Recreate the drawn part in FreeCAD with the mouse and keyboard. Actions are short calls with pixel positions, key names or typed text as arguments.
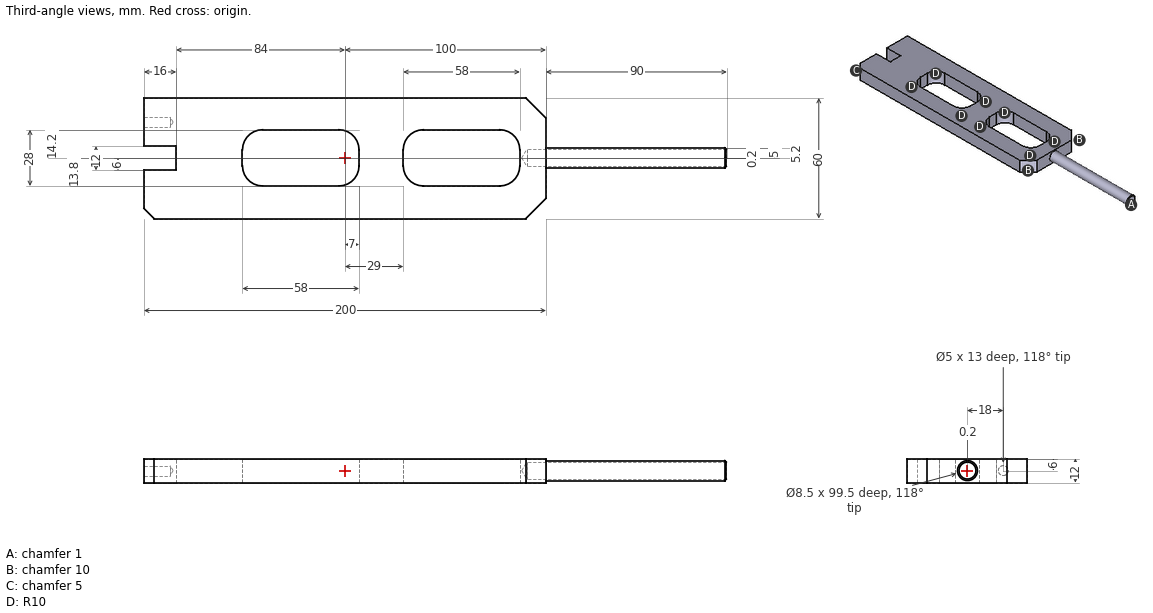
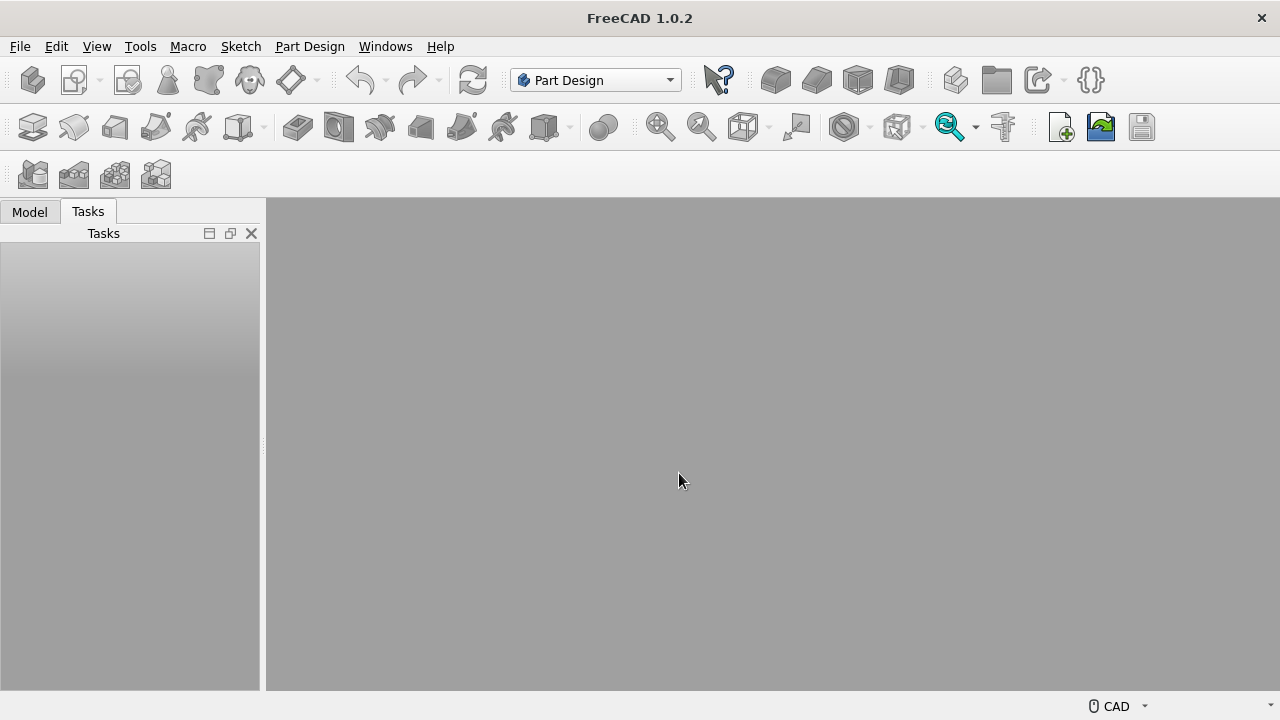
key(ctrl+n)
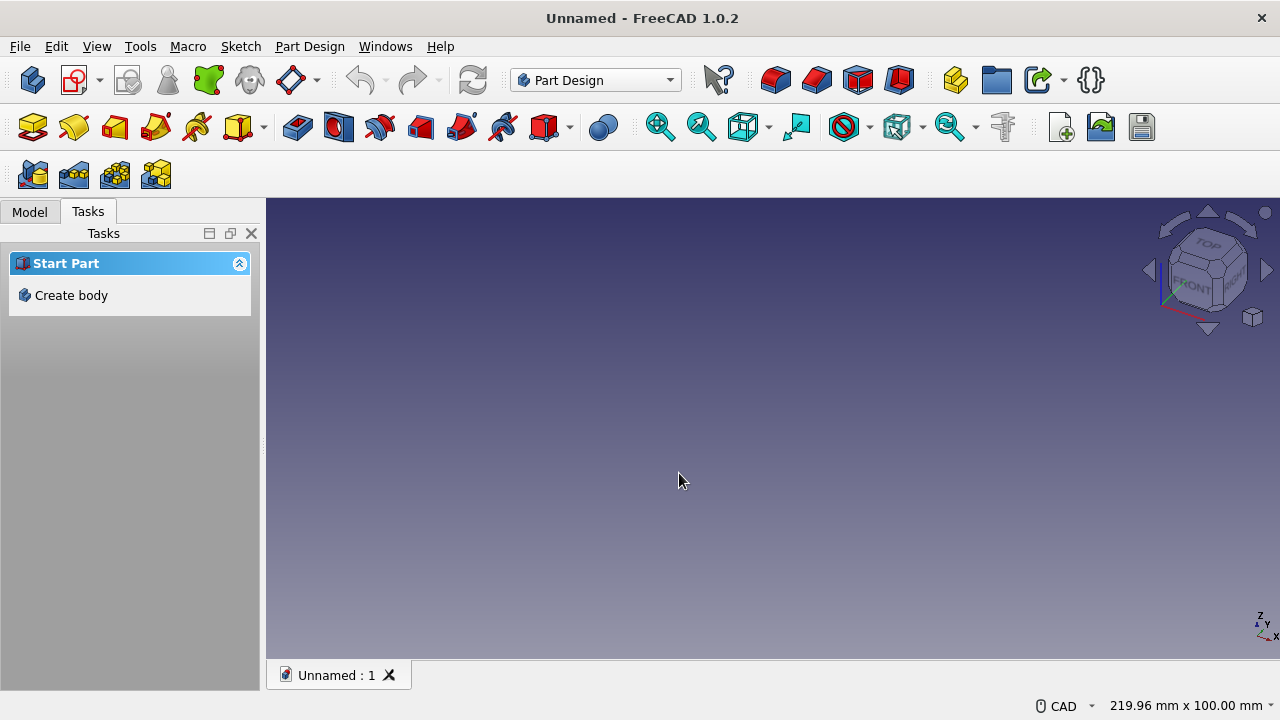
click(33, 80)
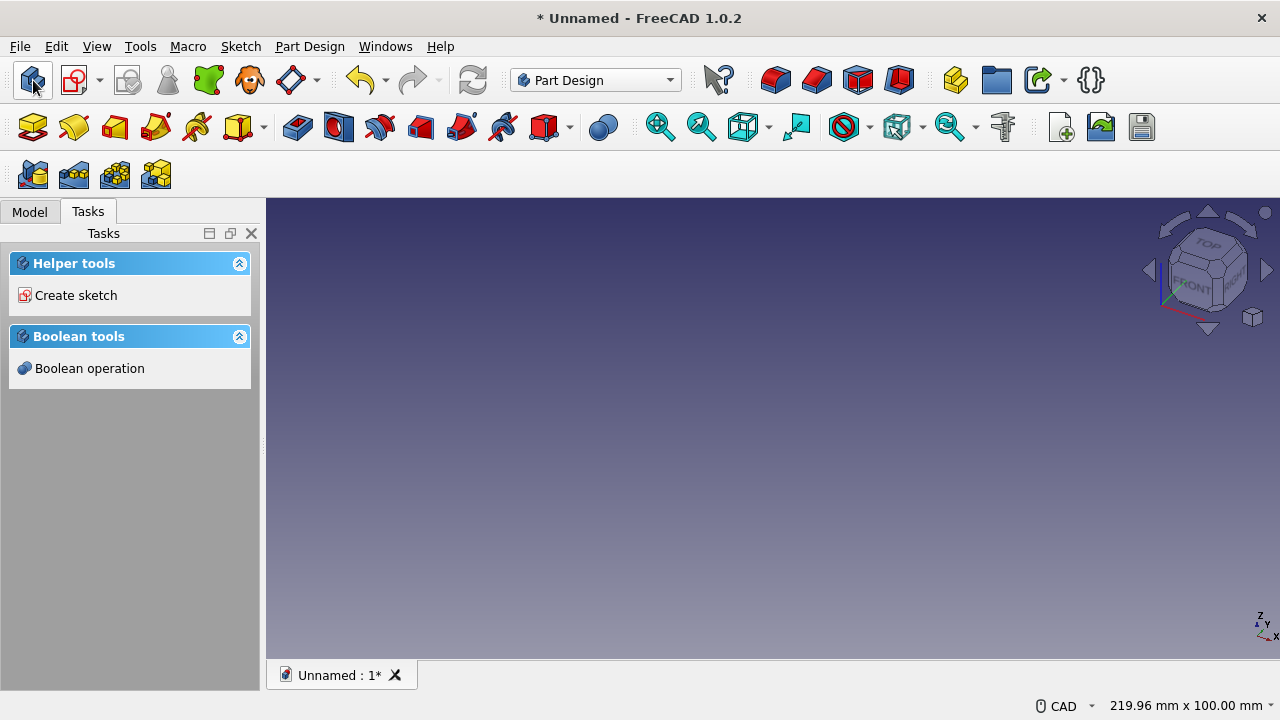
click(30, 212)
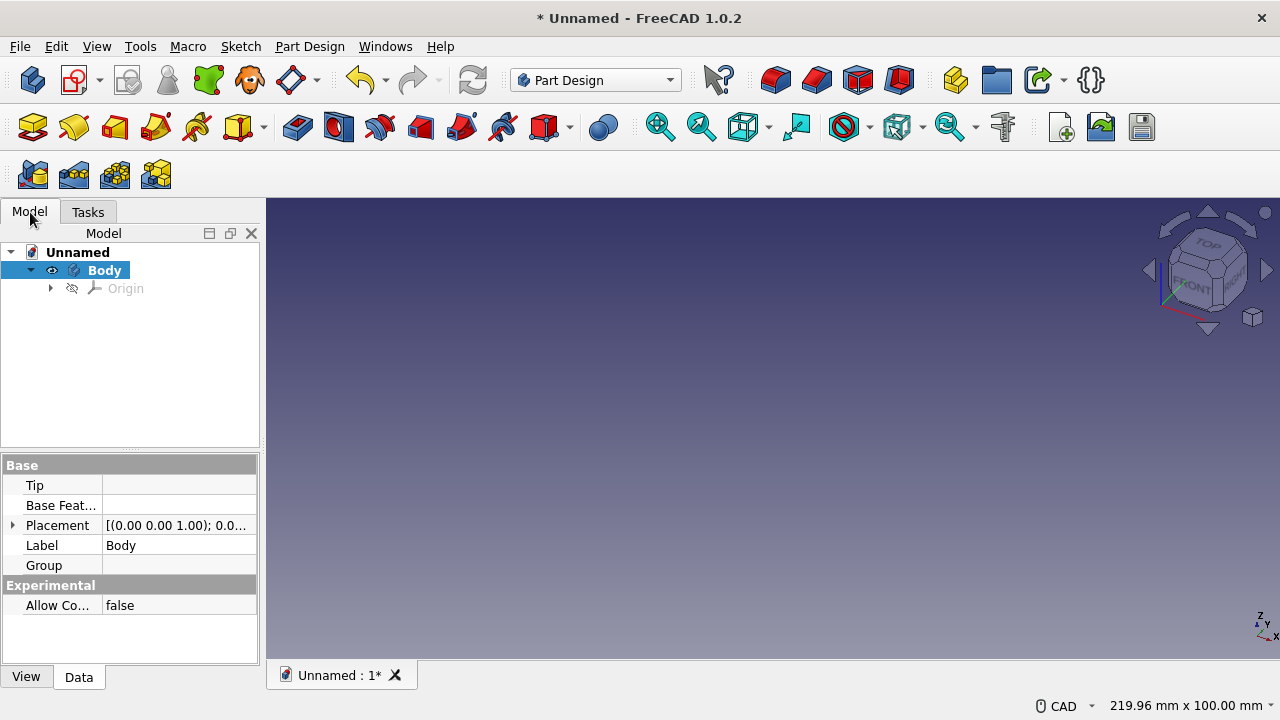
click(51, 288)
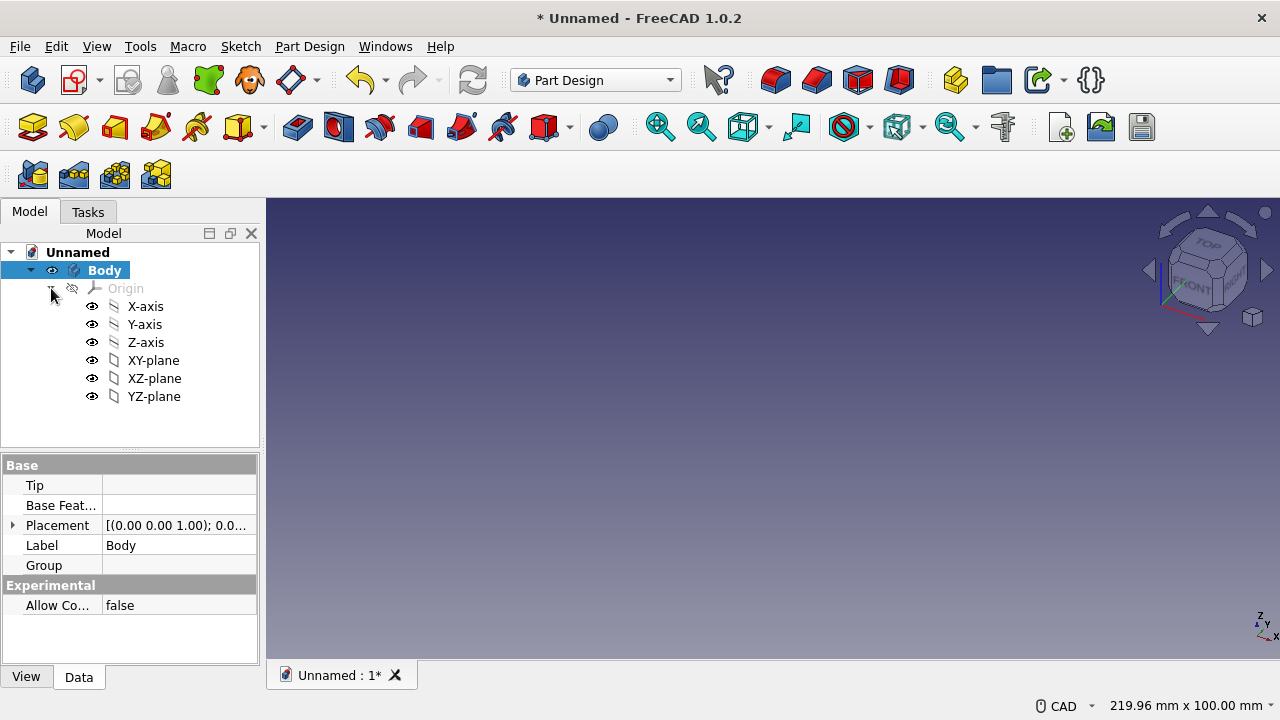
click(137, 360)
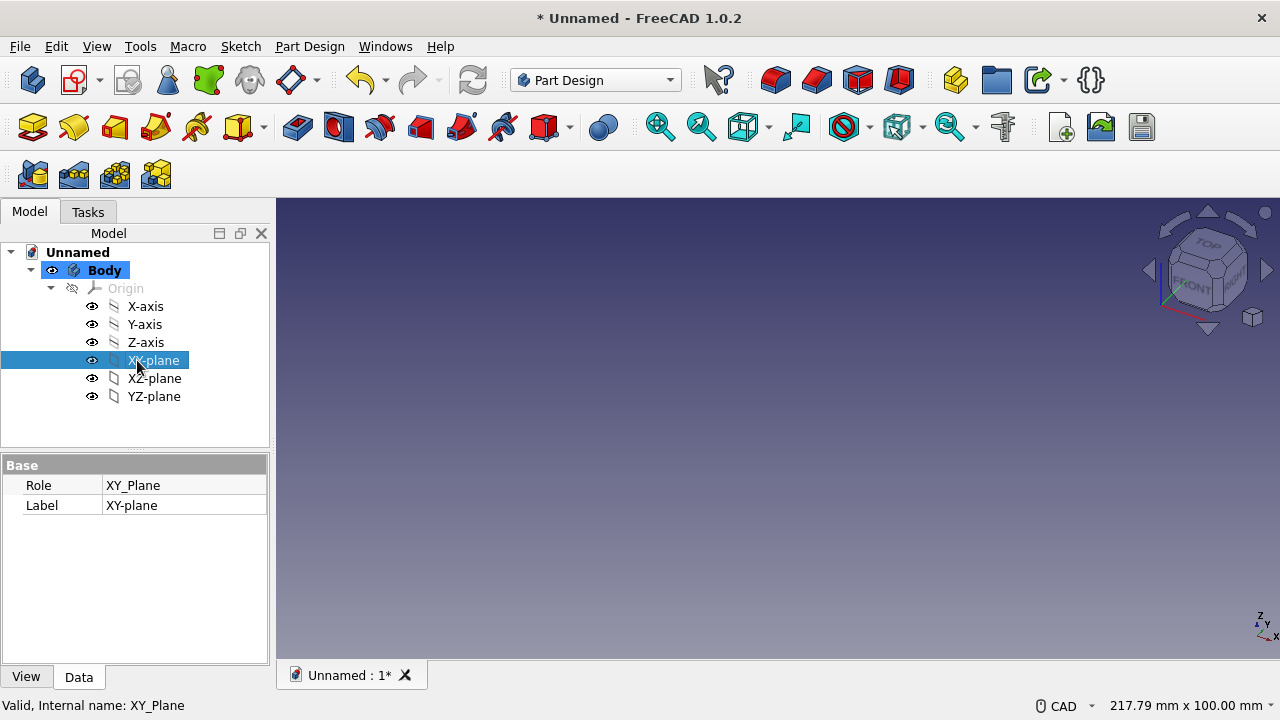
click(290, 80)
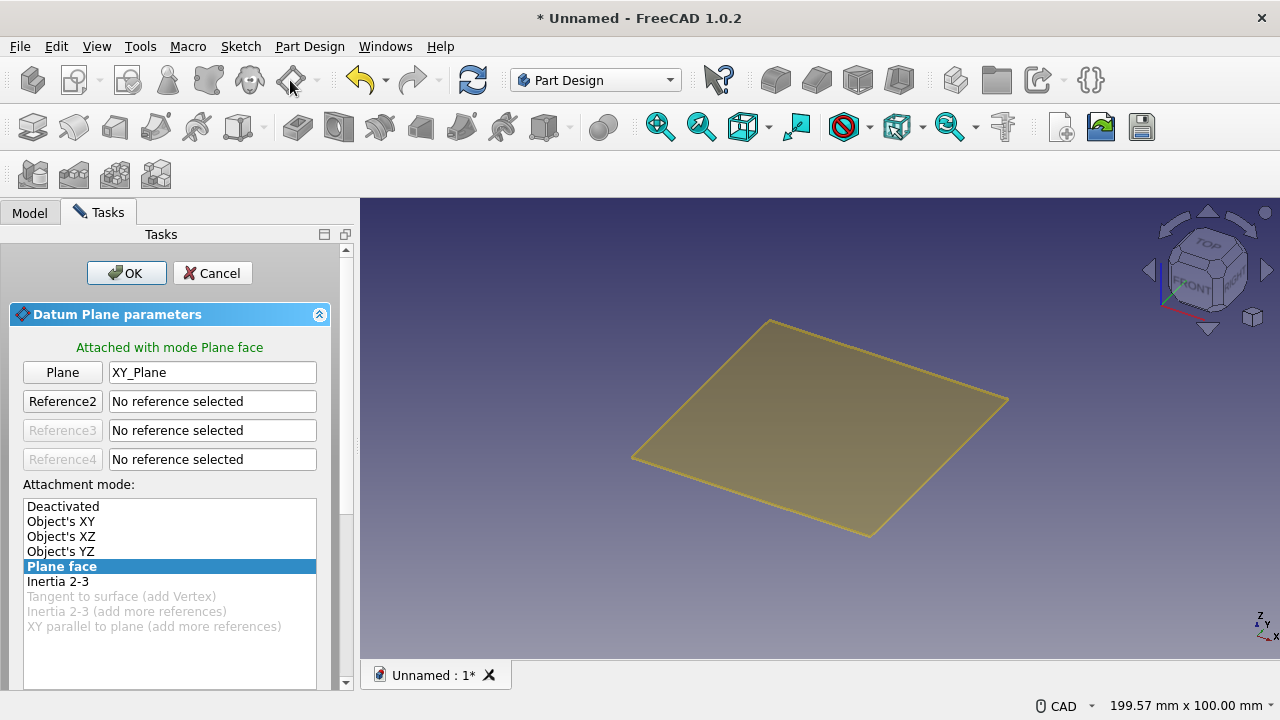
scroll(346, 467, down, 4)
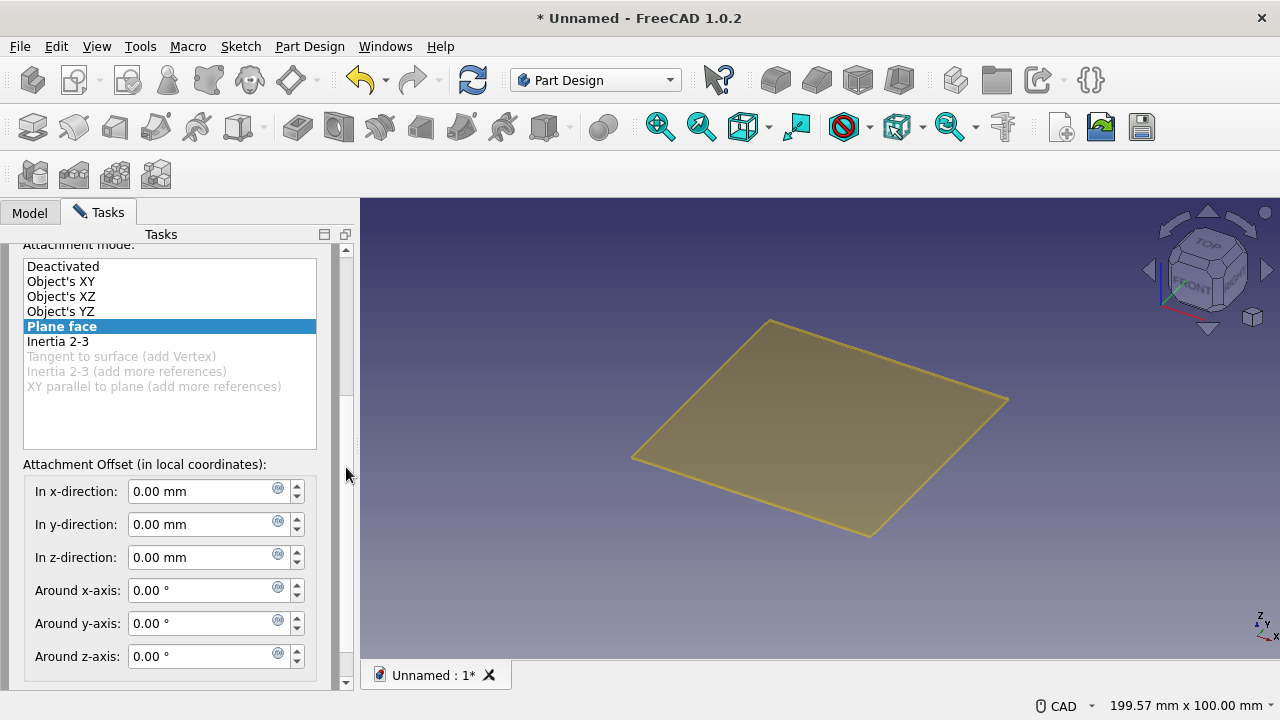
triple_click(210, 558)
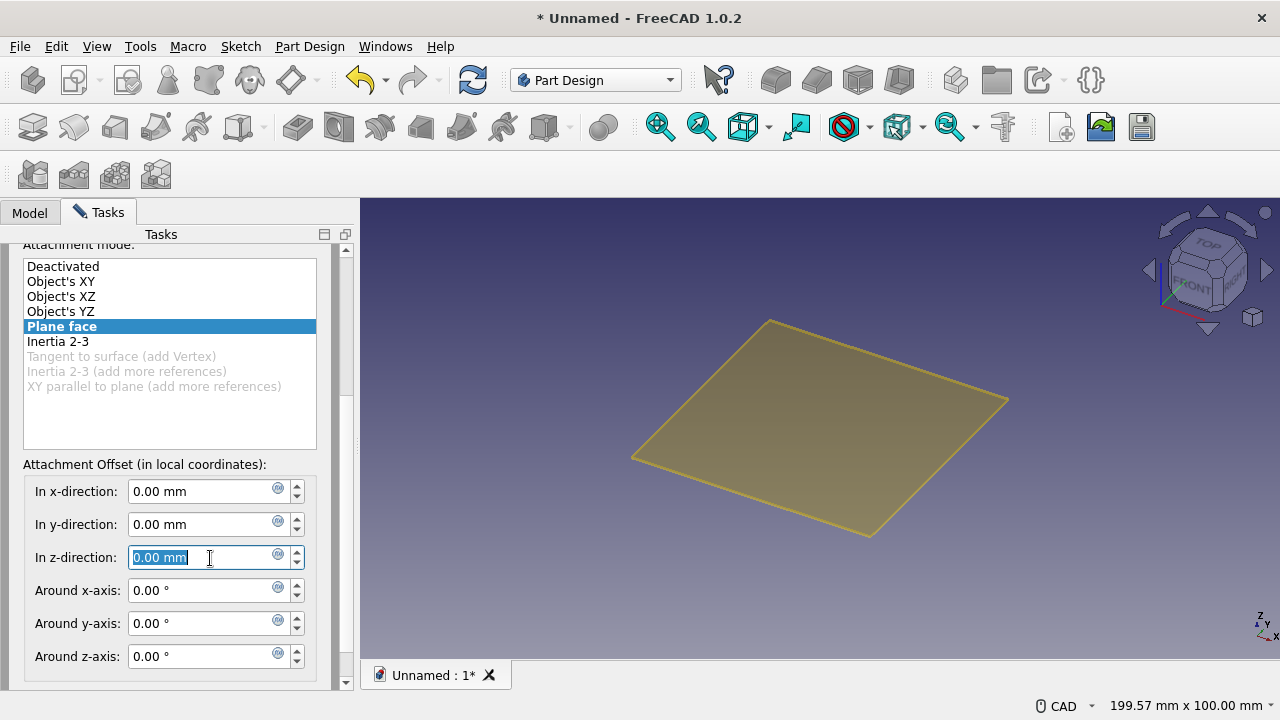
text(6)
key(Tab)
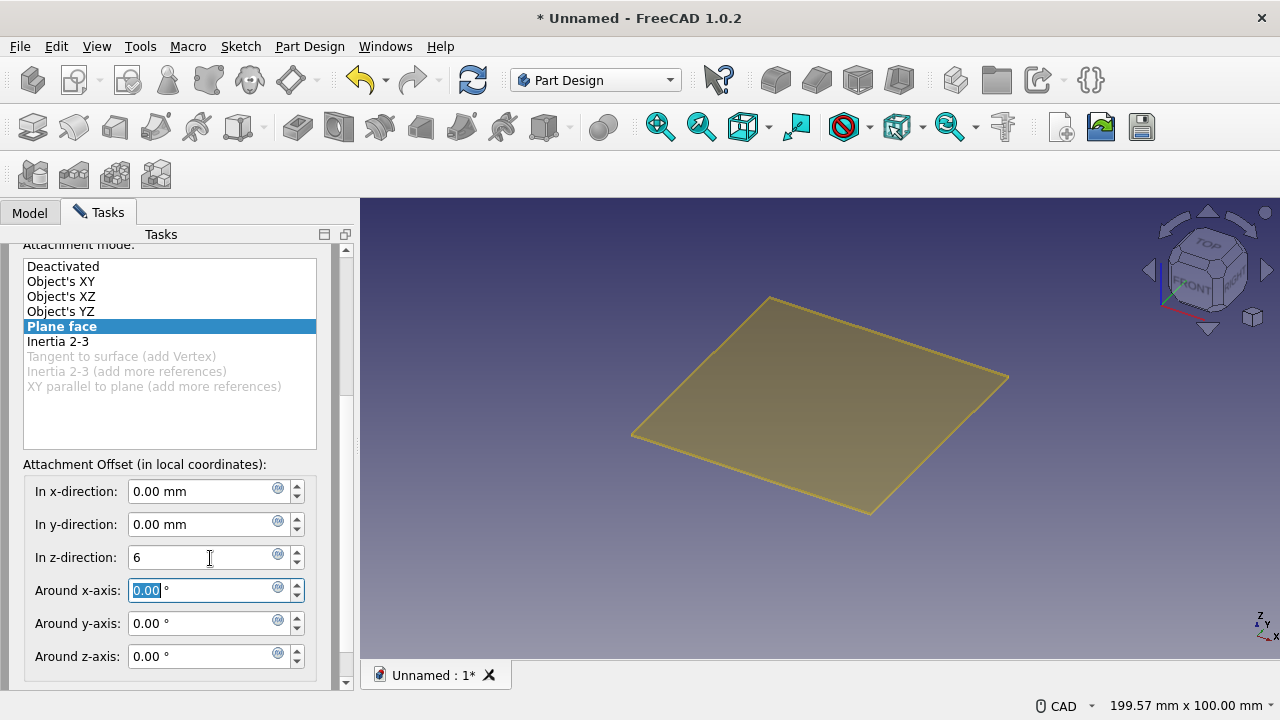
scroll(346, 467, up, 5)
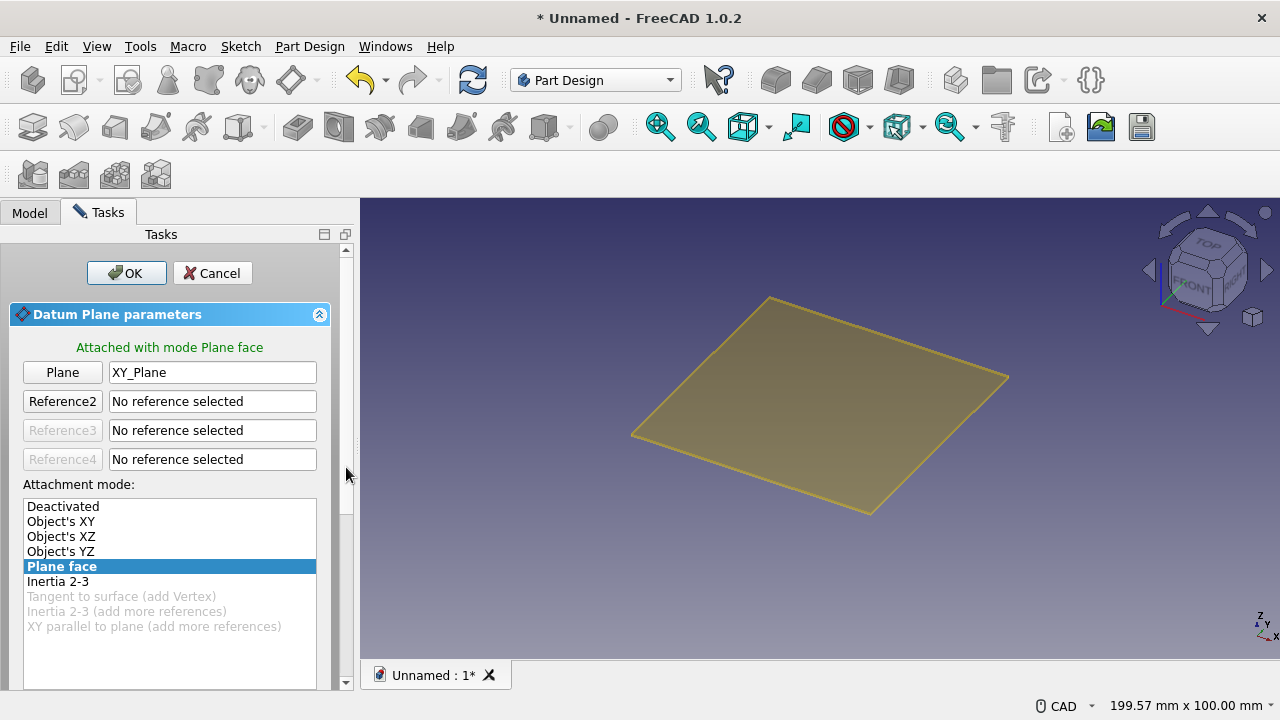
click(127, 273)